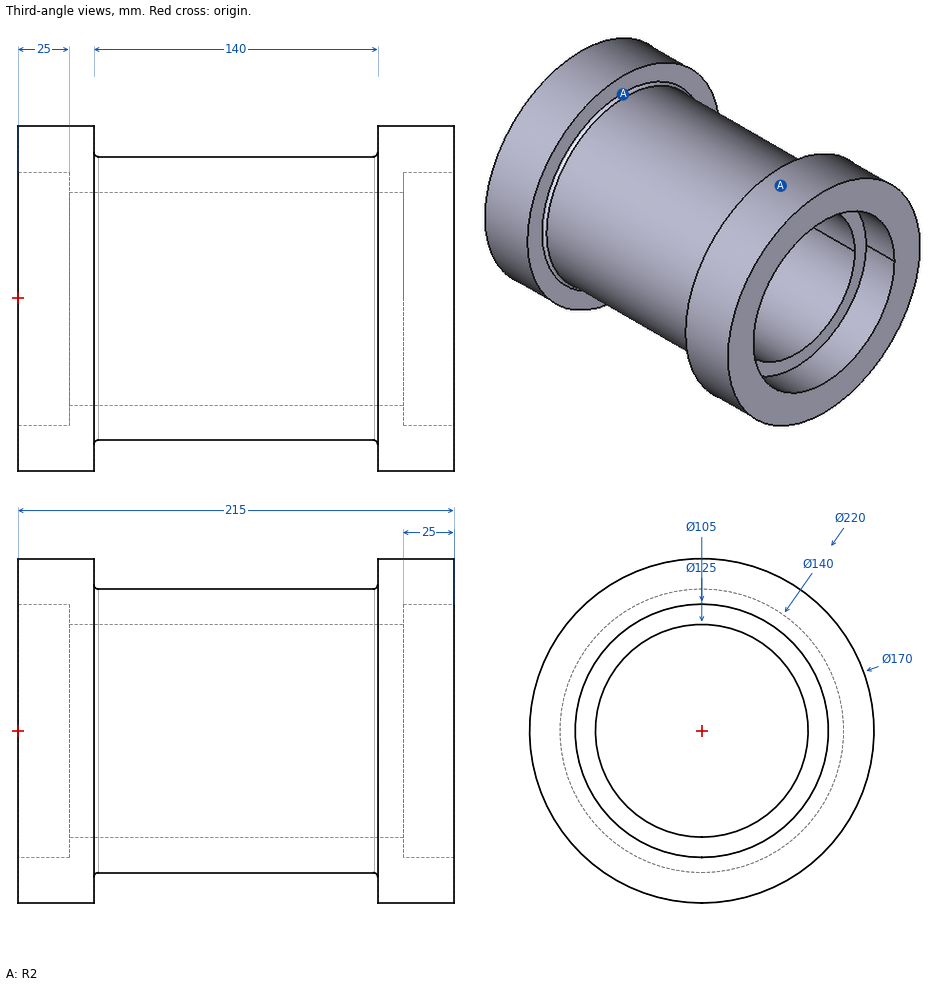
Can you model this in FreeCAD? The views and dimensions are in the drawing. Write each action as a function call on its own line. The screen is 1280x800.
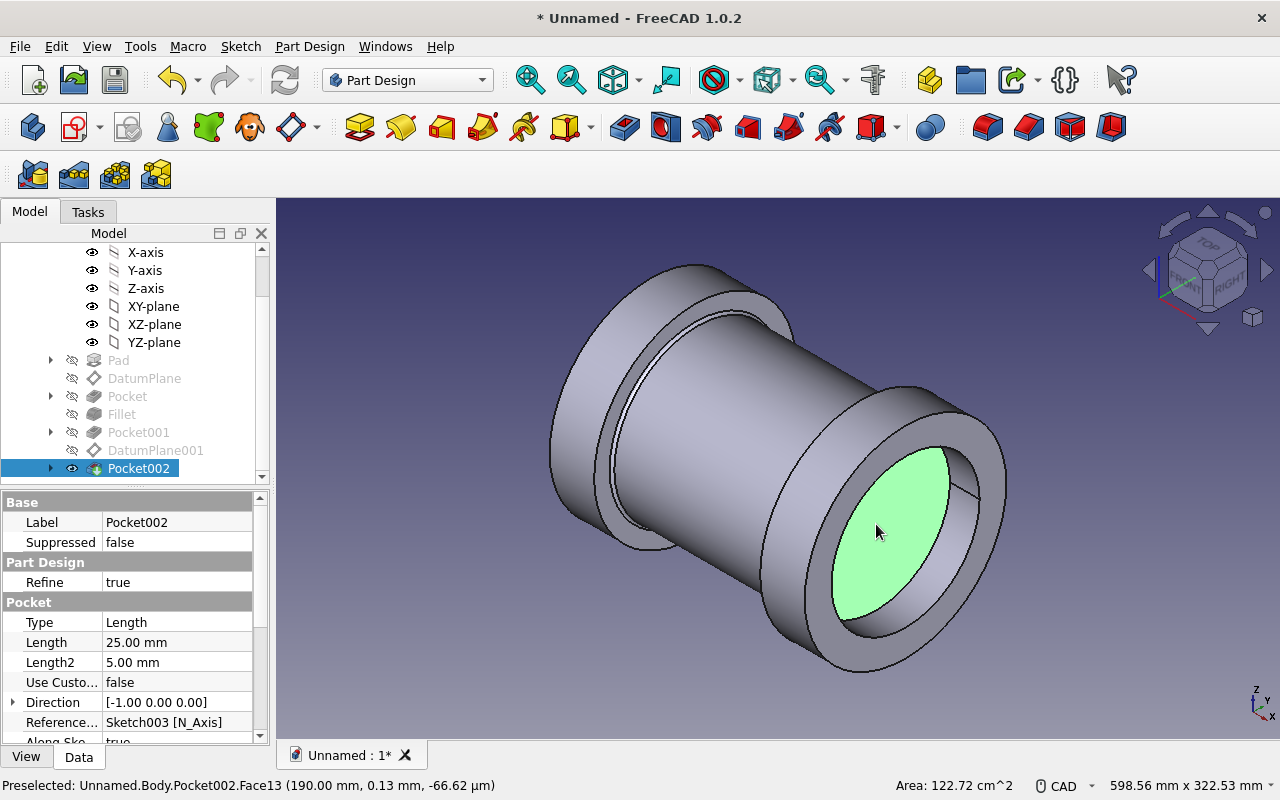
click(74, 128)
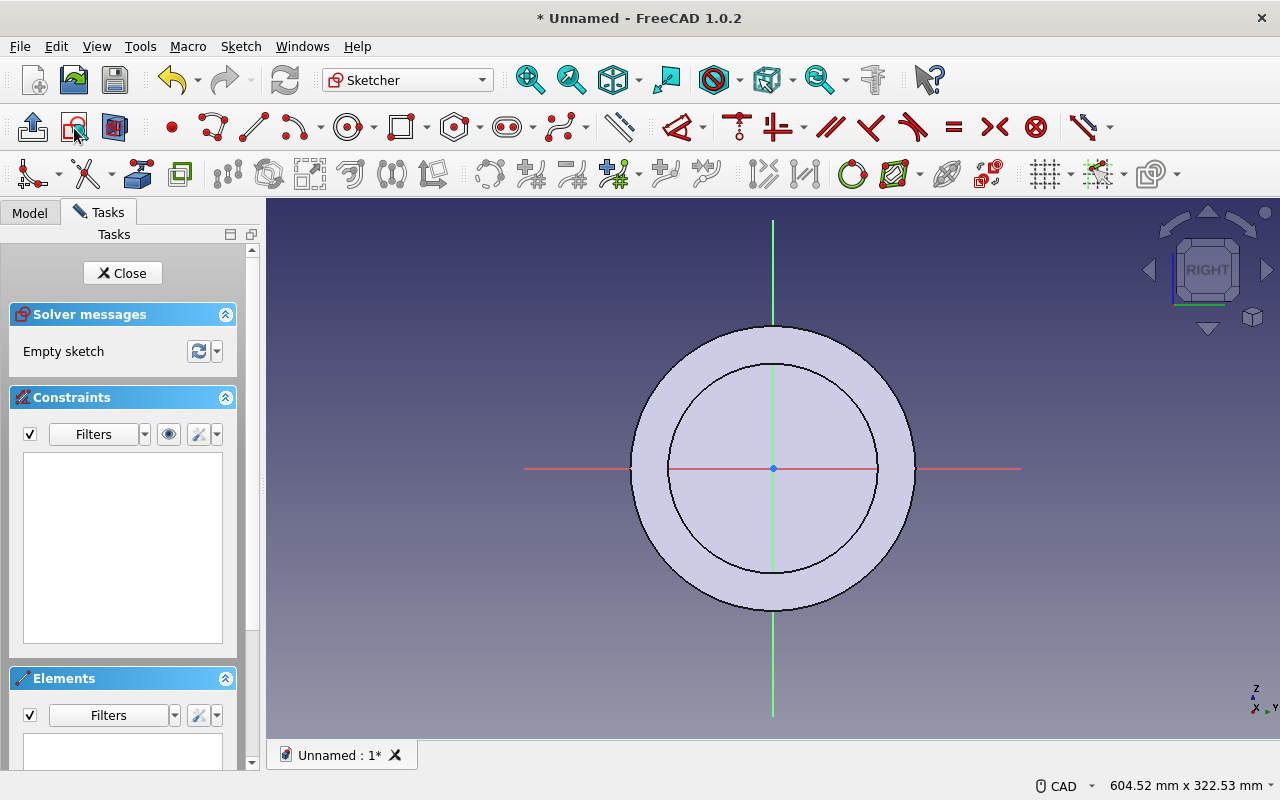
scroll(856, 468, up, 3)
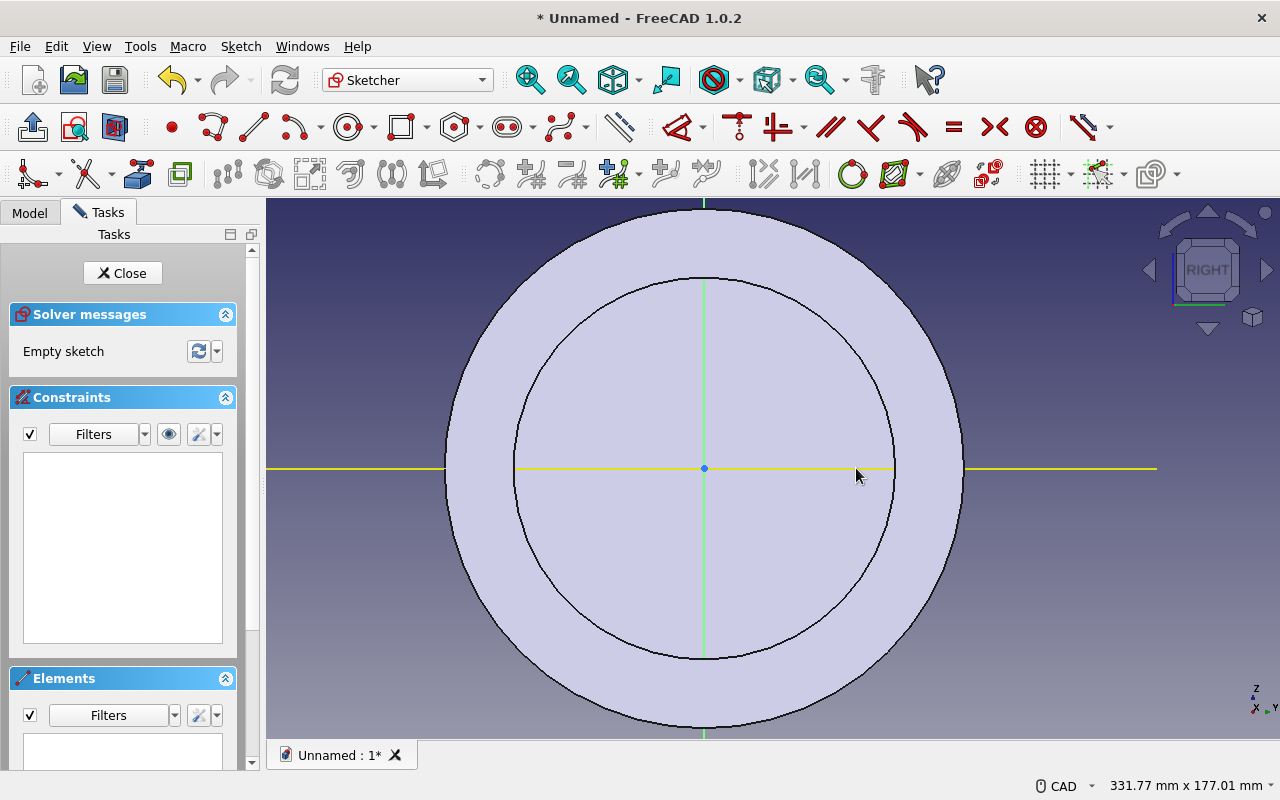
key(g)
key(c)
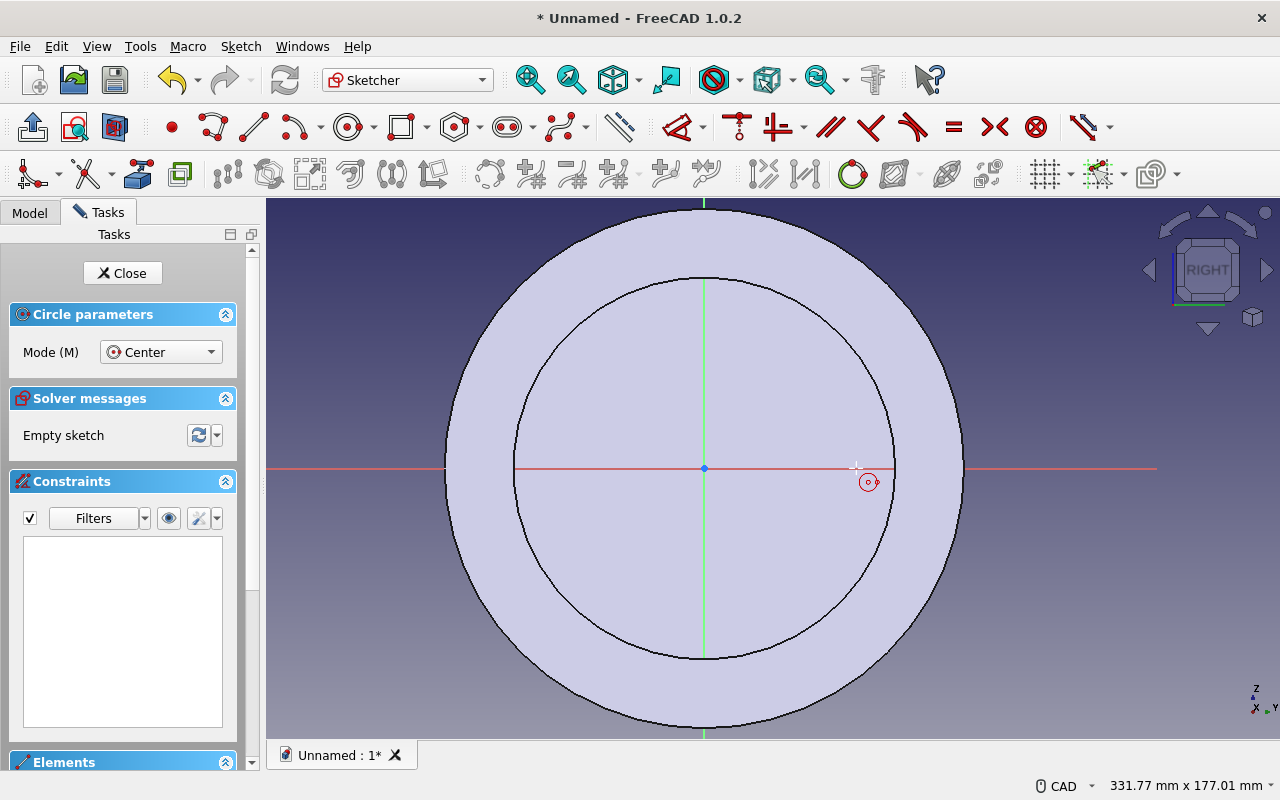
click(704, 468)
move(818, 355)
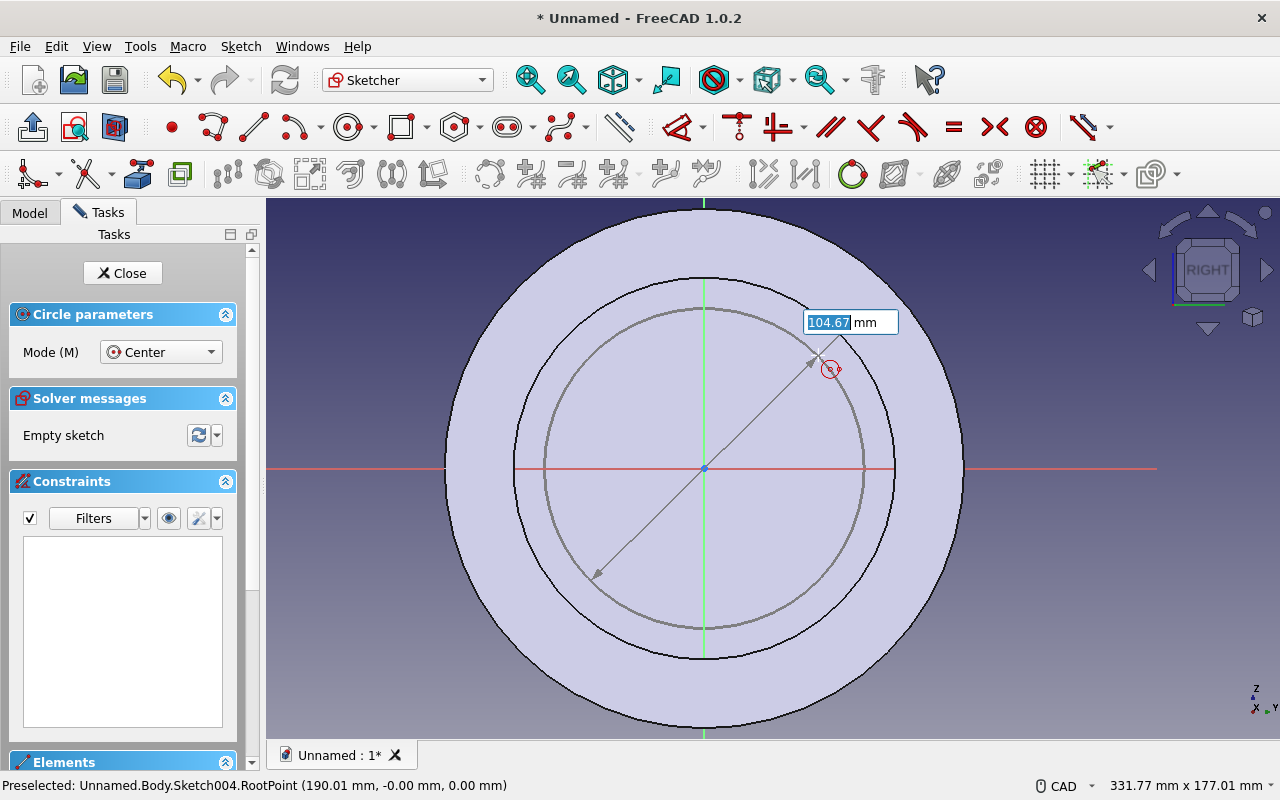
text(105)
key(Return)
key(Escape)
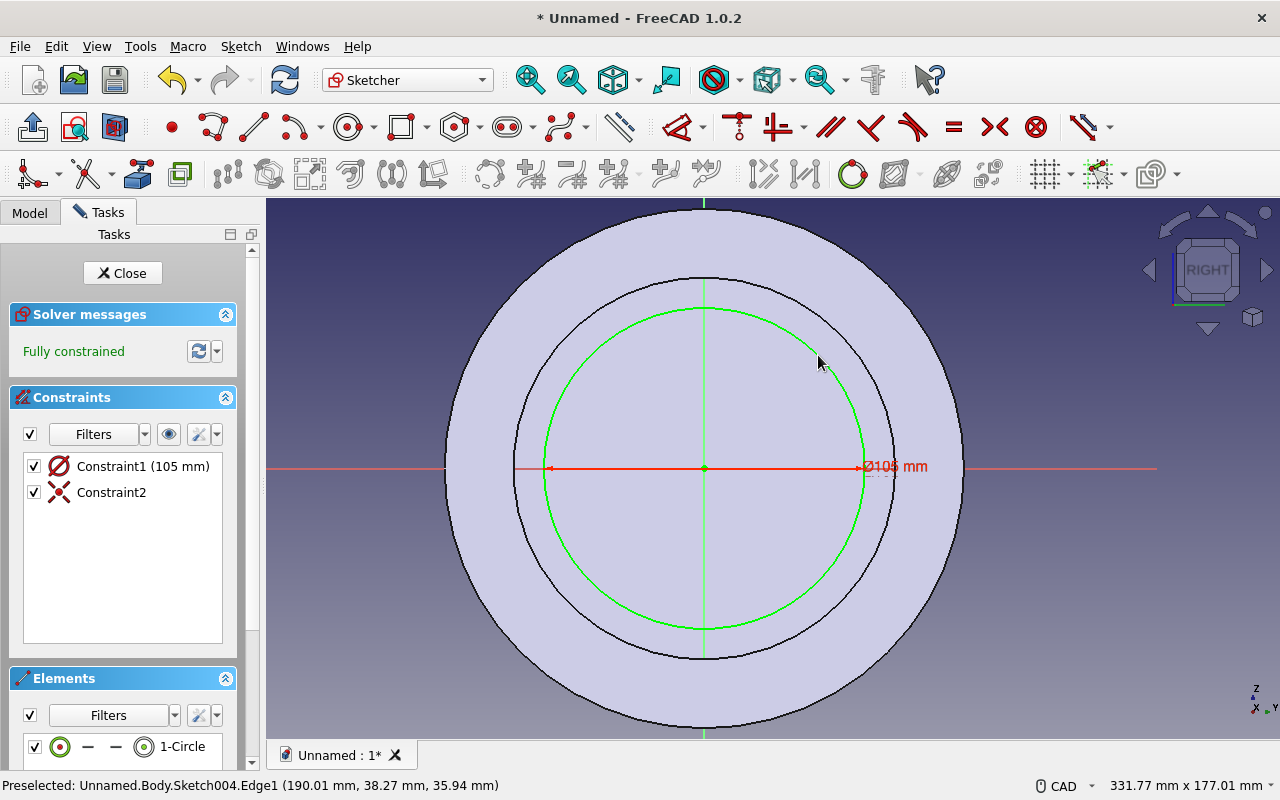
click(123, 273)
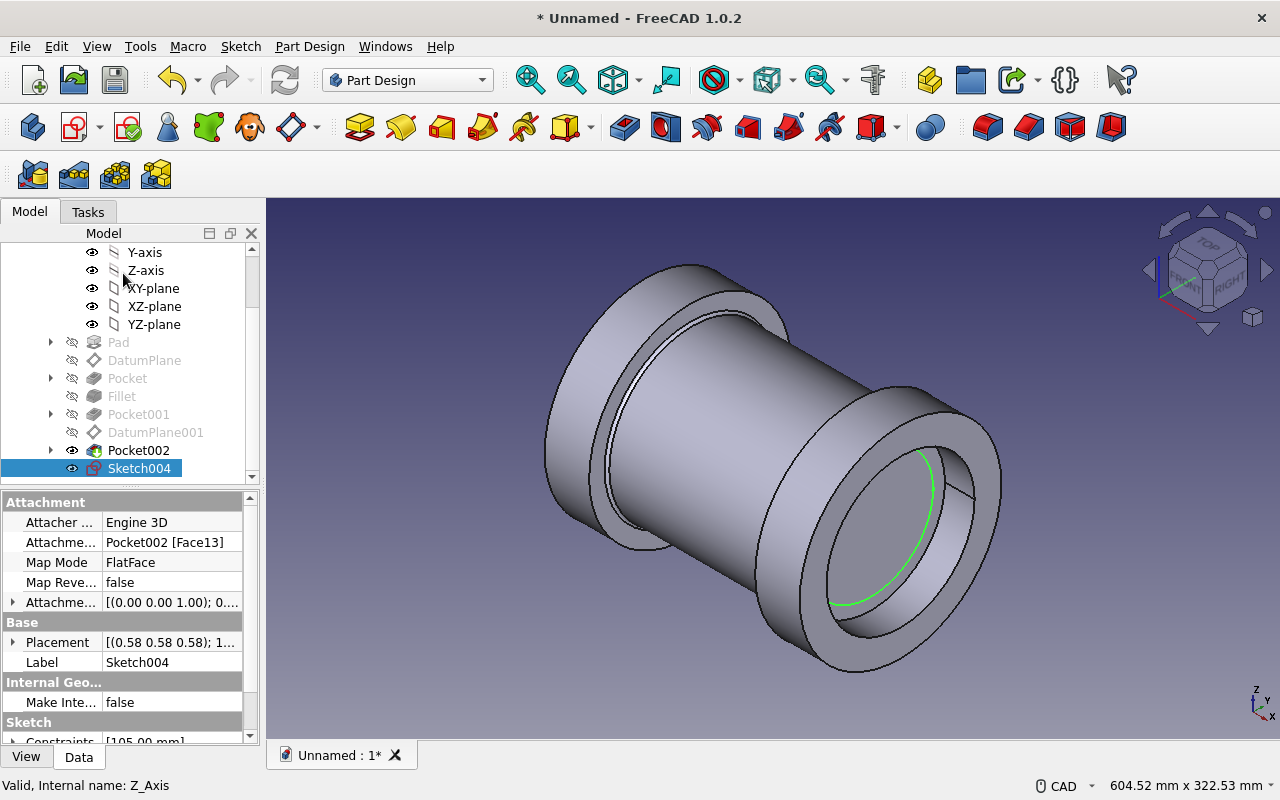
click(625, 128)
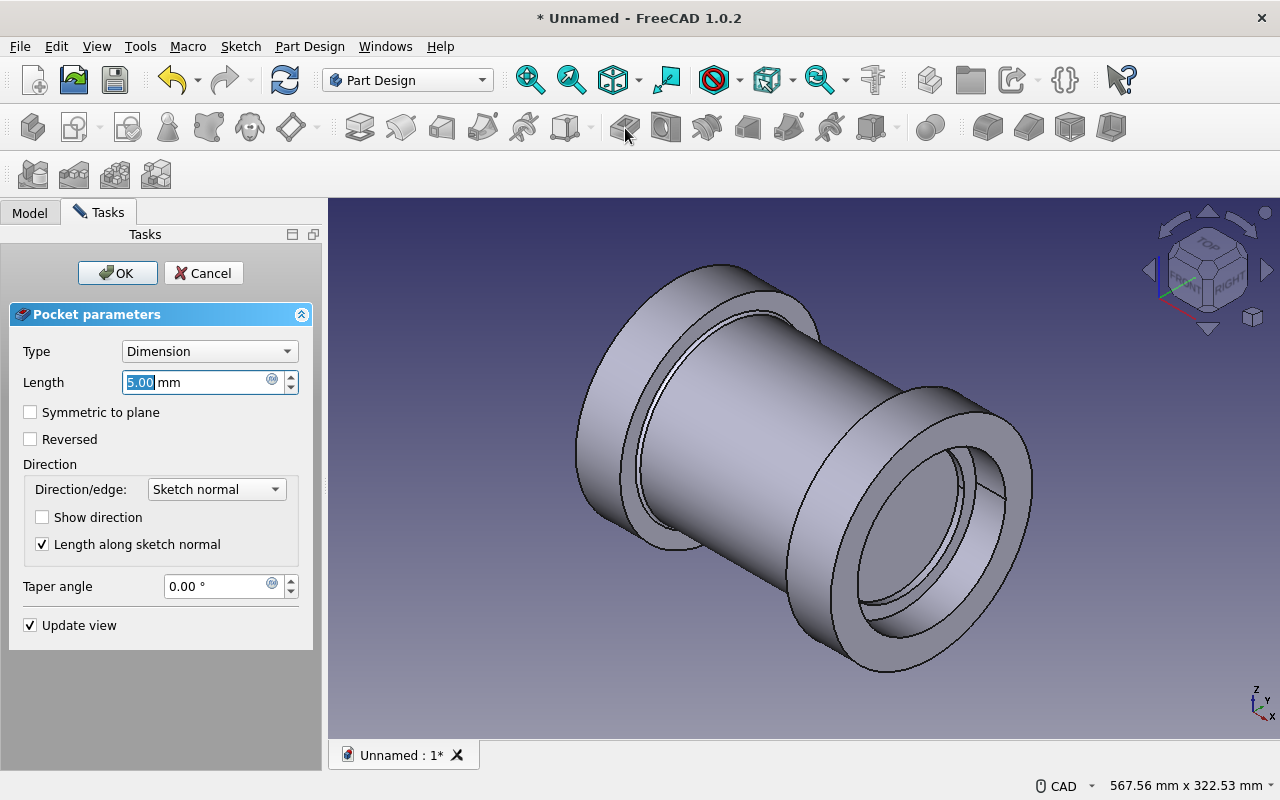
click(210, 352)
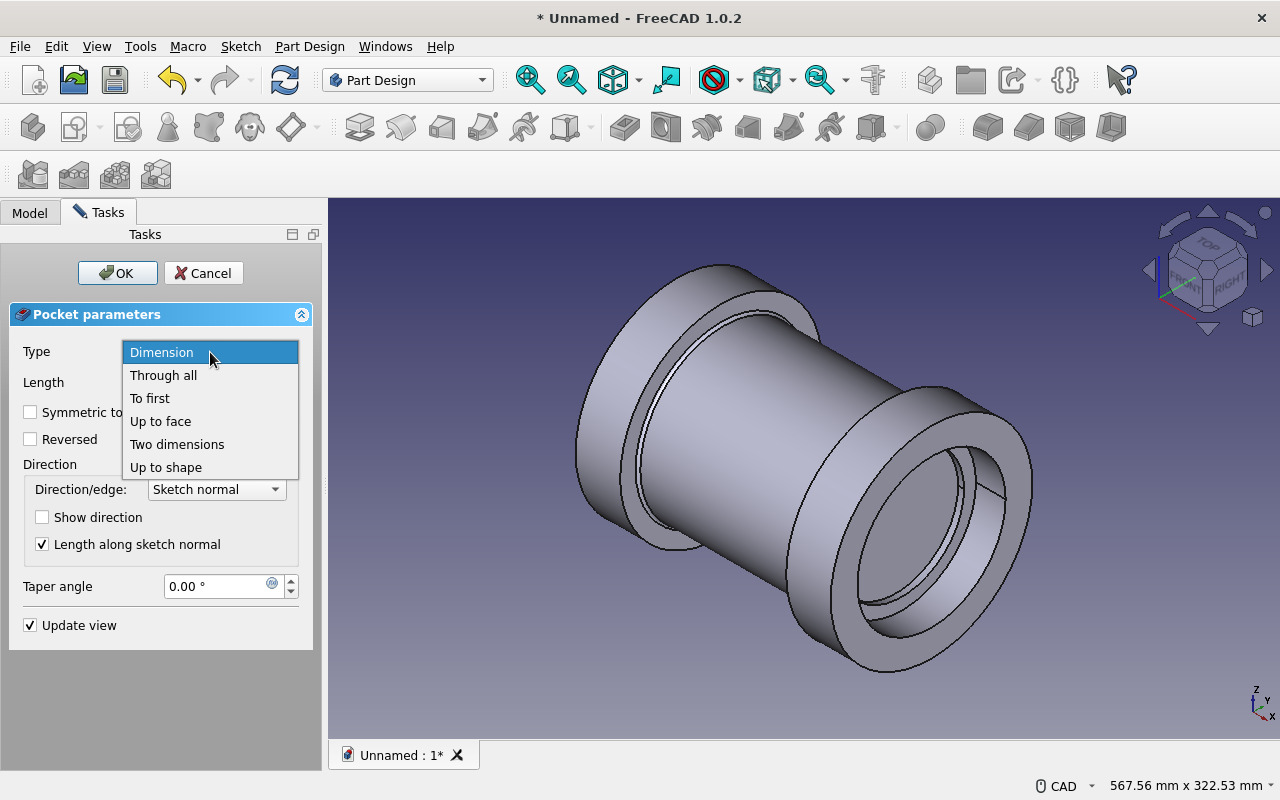
click(208, 376)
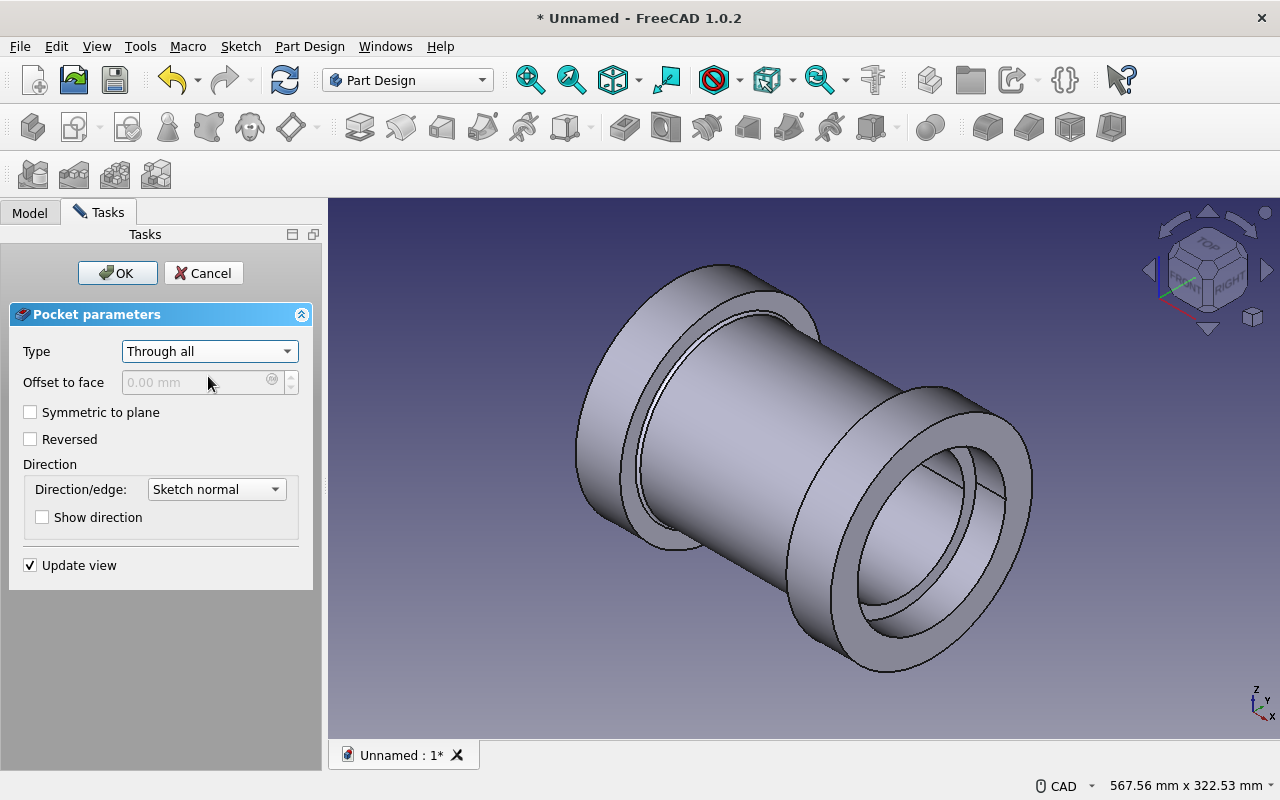
click(118, 273)